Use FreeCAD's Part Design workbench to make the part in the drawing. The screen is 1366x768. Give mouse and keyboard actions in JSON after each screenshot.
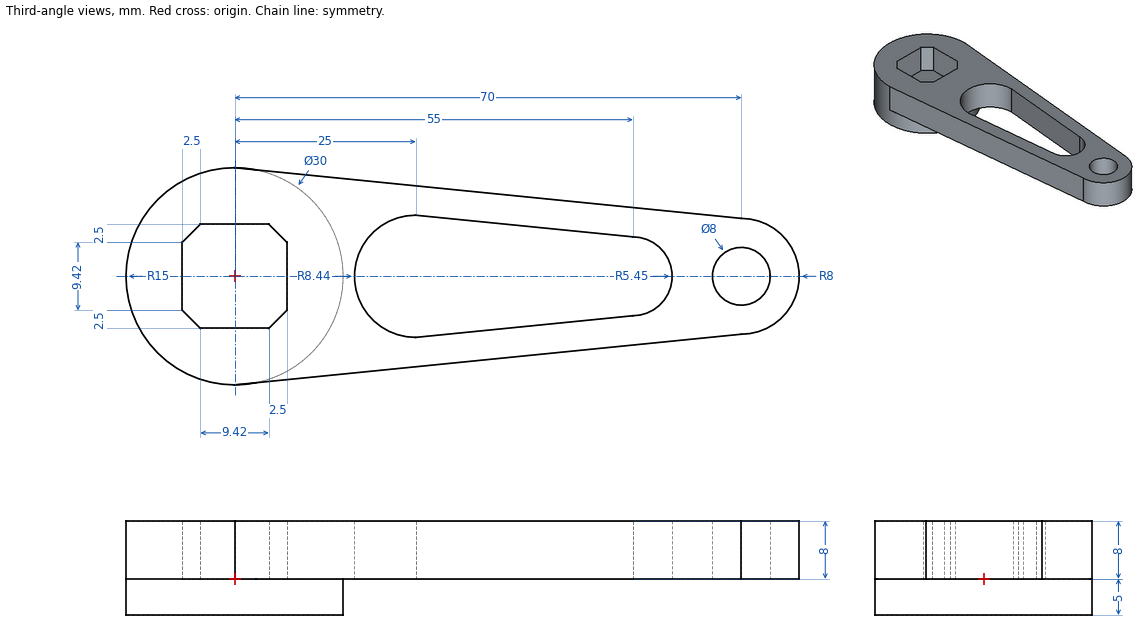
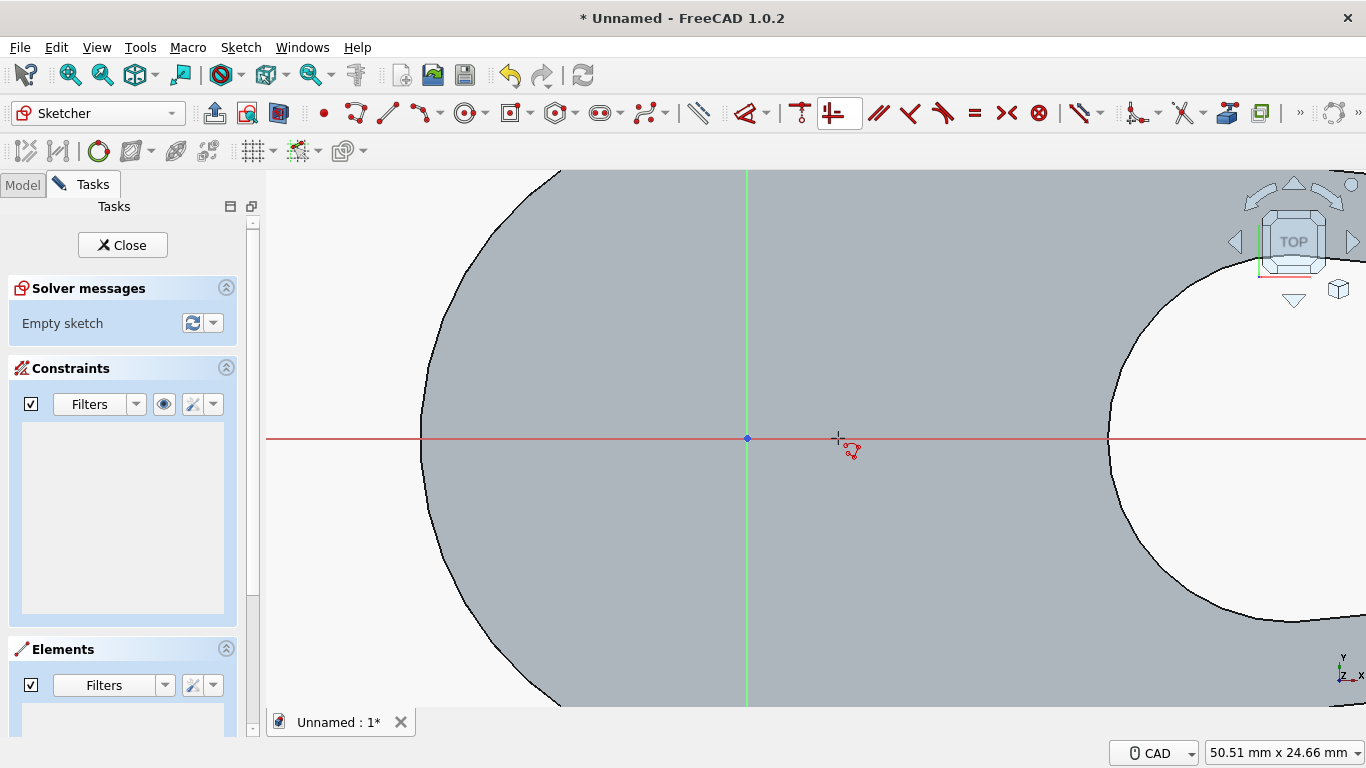
{"action": "left_click", "coordinate": [645, 281]}
{"action": "left_click", "coordinate": [590, 336]}
{"action": "left_click", "coordinate": [590, 541]}
{"action": "left_click", "coordinate": [645, 596]}
{"action": "left_click", "coordinate": [850, 596]}
{"action": "left_click", "coordinate": [904, 541]}
{"action": "left_click", "coordinate": [904, 336]}
{"action": "left_click", "coordinate": [850, 281]}
{"action": "left_click", "coordinate": [645, 282]}
{"action": "key", "text": "Escape"}
{"action": "key", "text": "Escape"}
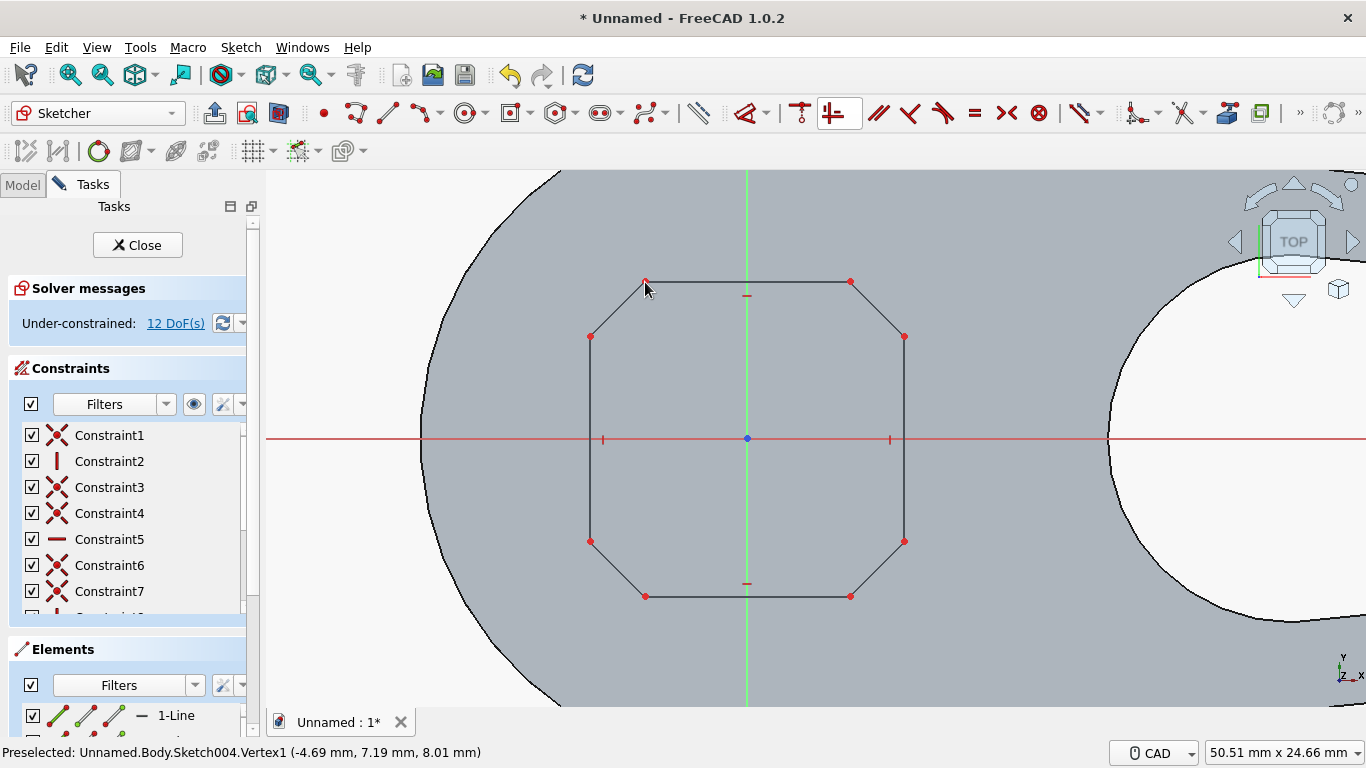
{"action": "left_click", "coordinate": [645, 282]}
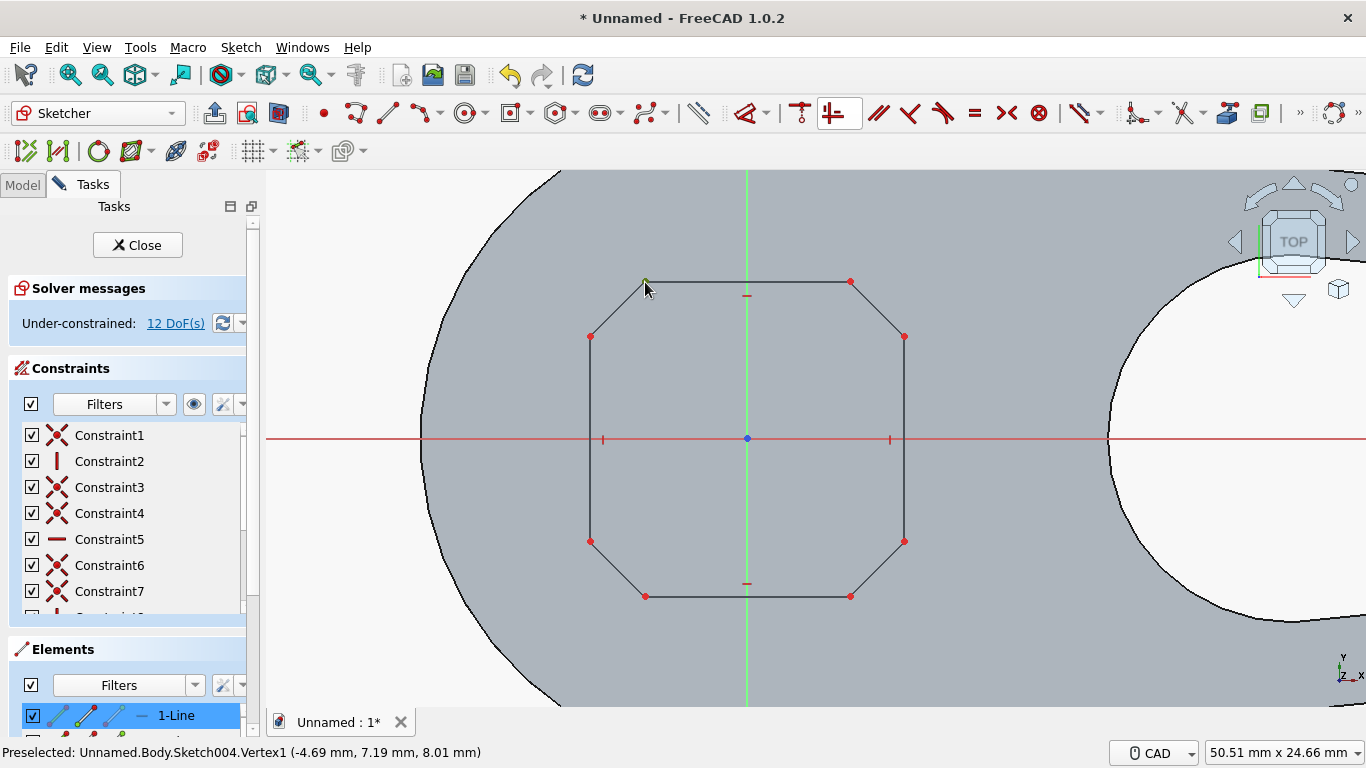
{"action": "left_click", "coordinate": [645, 597]}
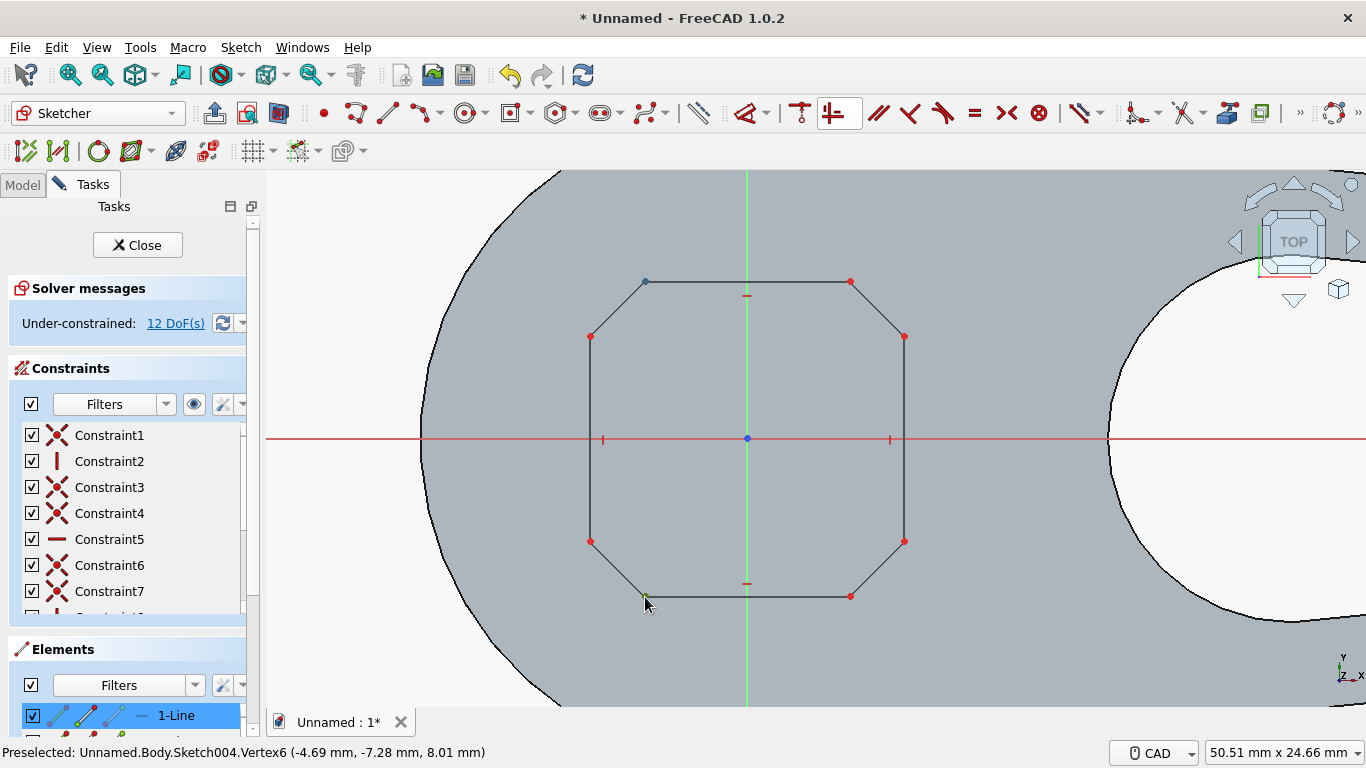
{"action": "left_click", "coordinate": [359, 438]}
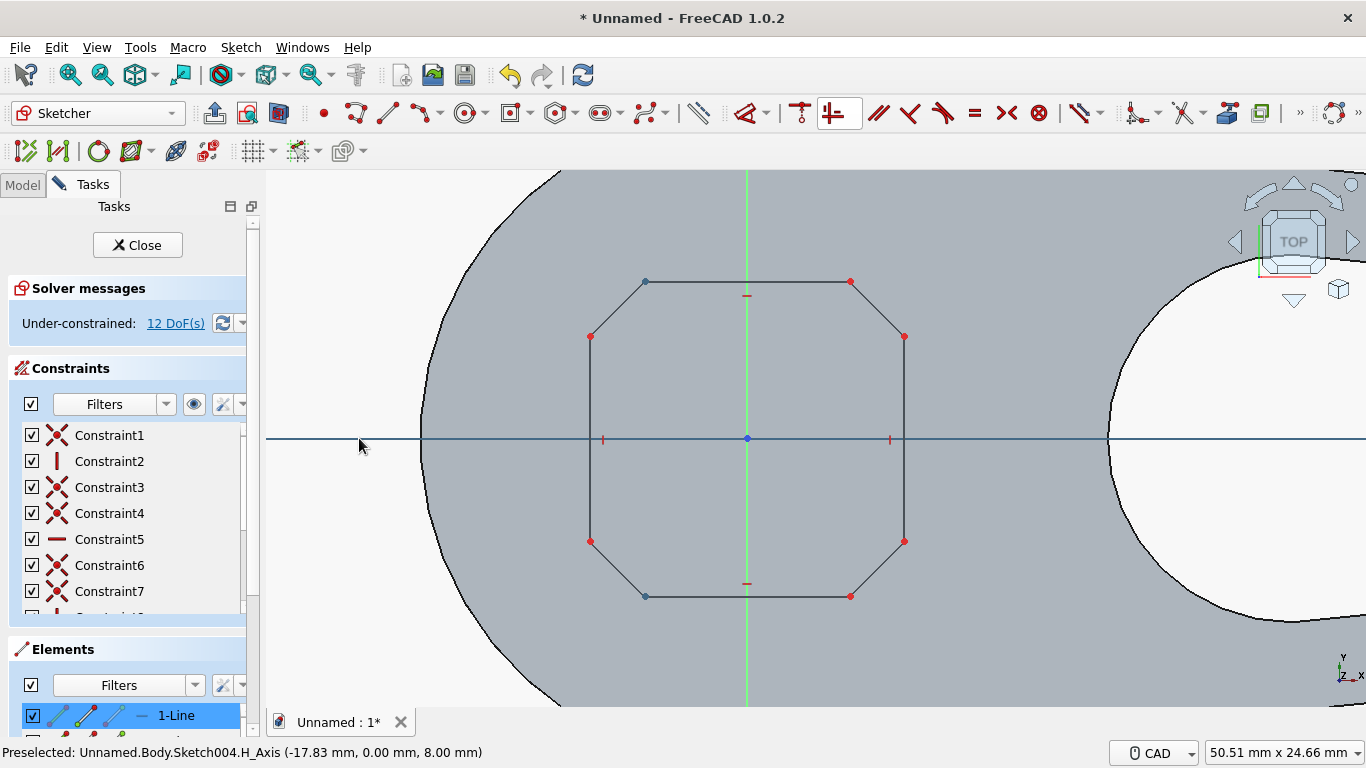
{"action": "key", "text": "s"}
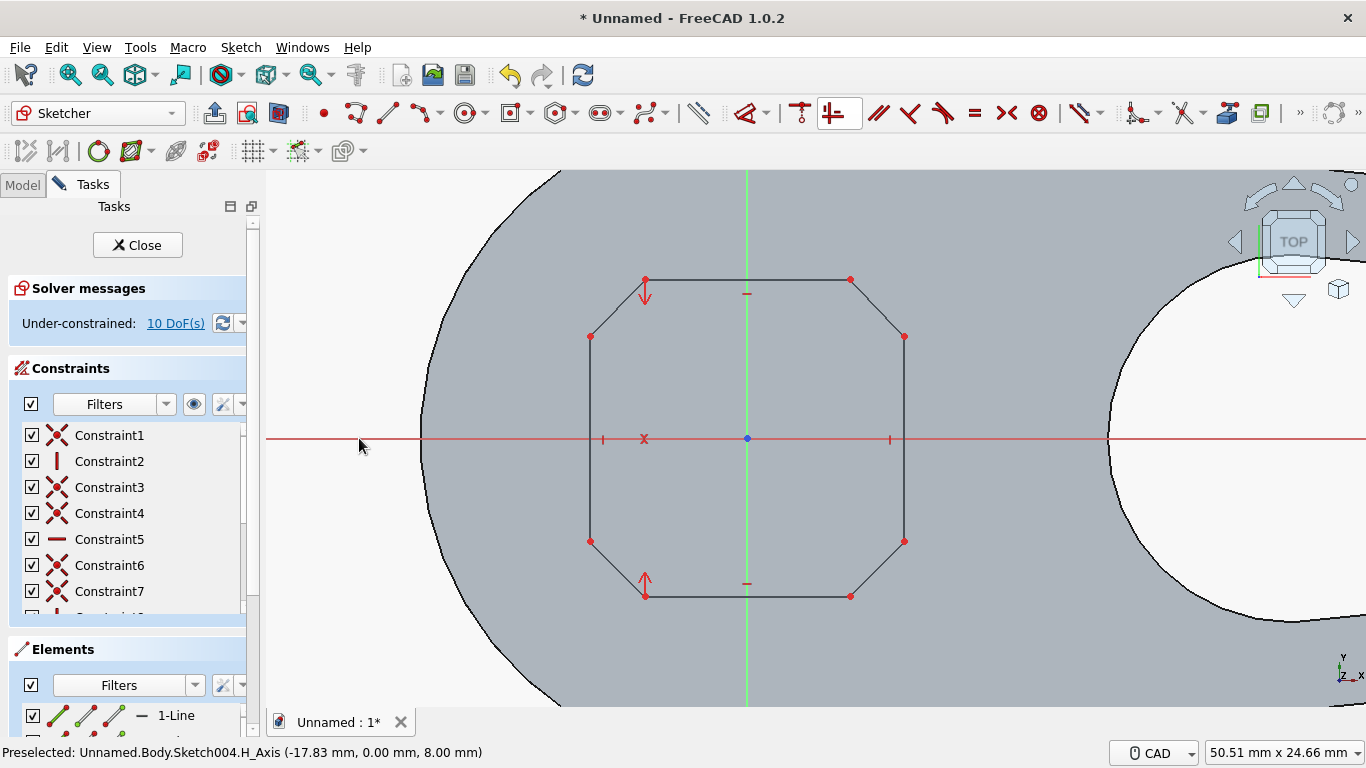
{"action": "left_click", "coordinate": [590, 542]}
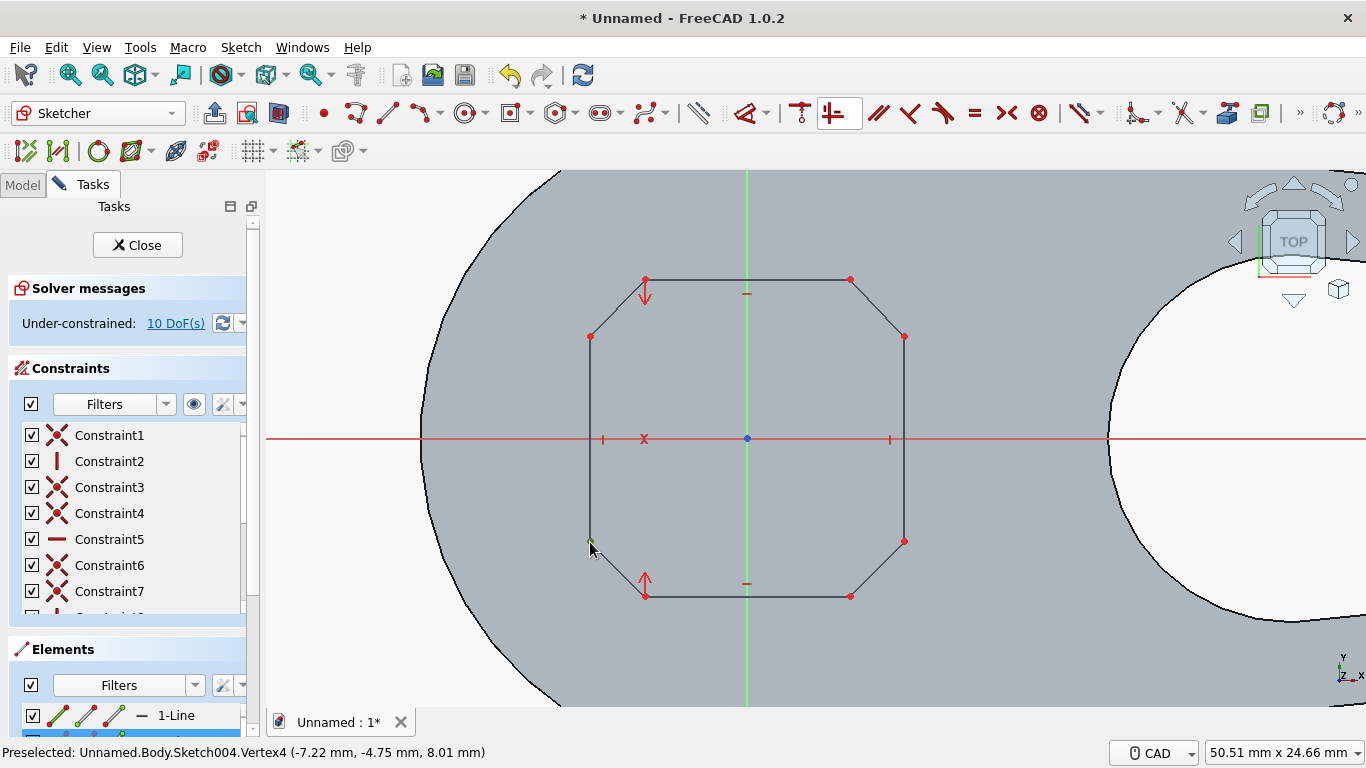
{"action": "left_click", "coordinate": [904, 542]}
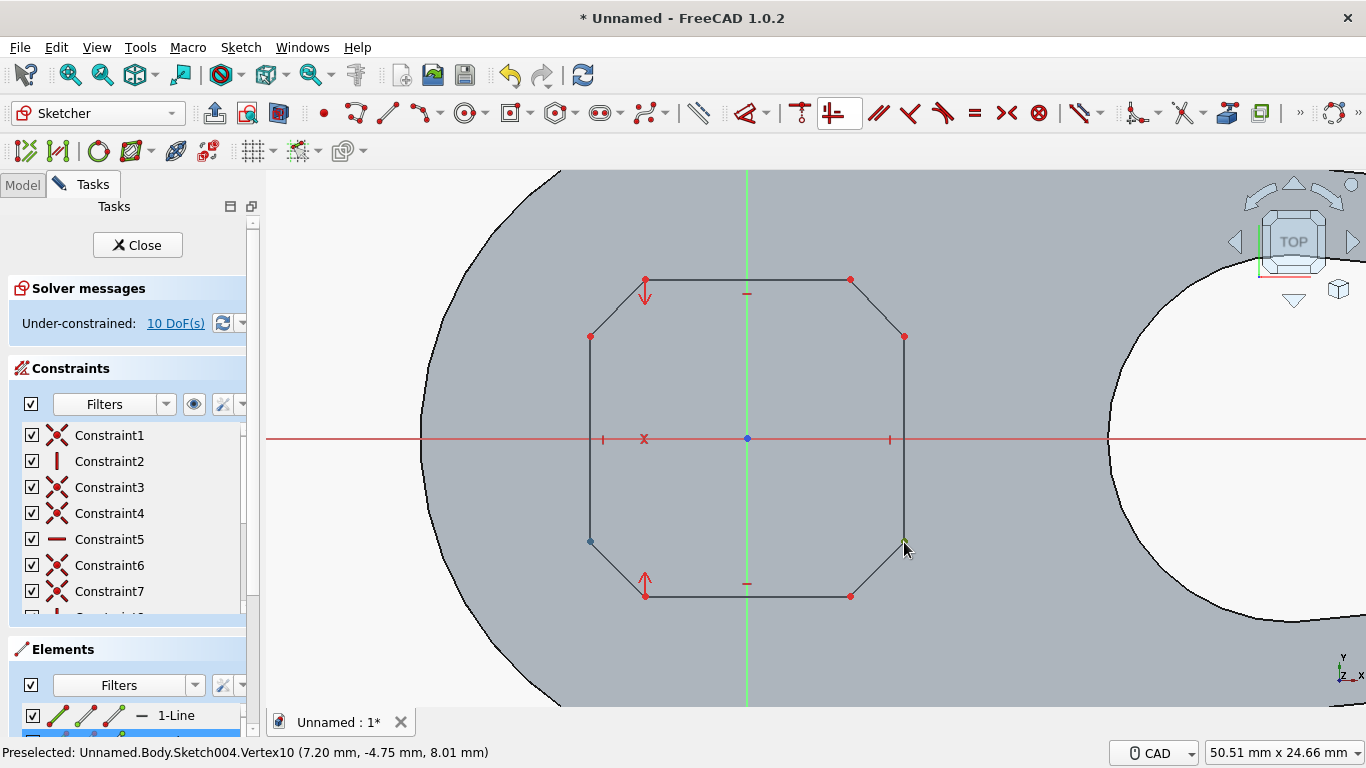
{"action": "left_click", "coordinate": [747, 645]}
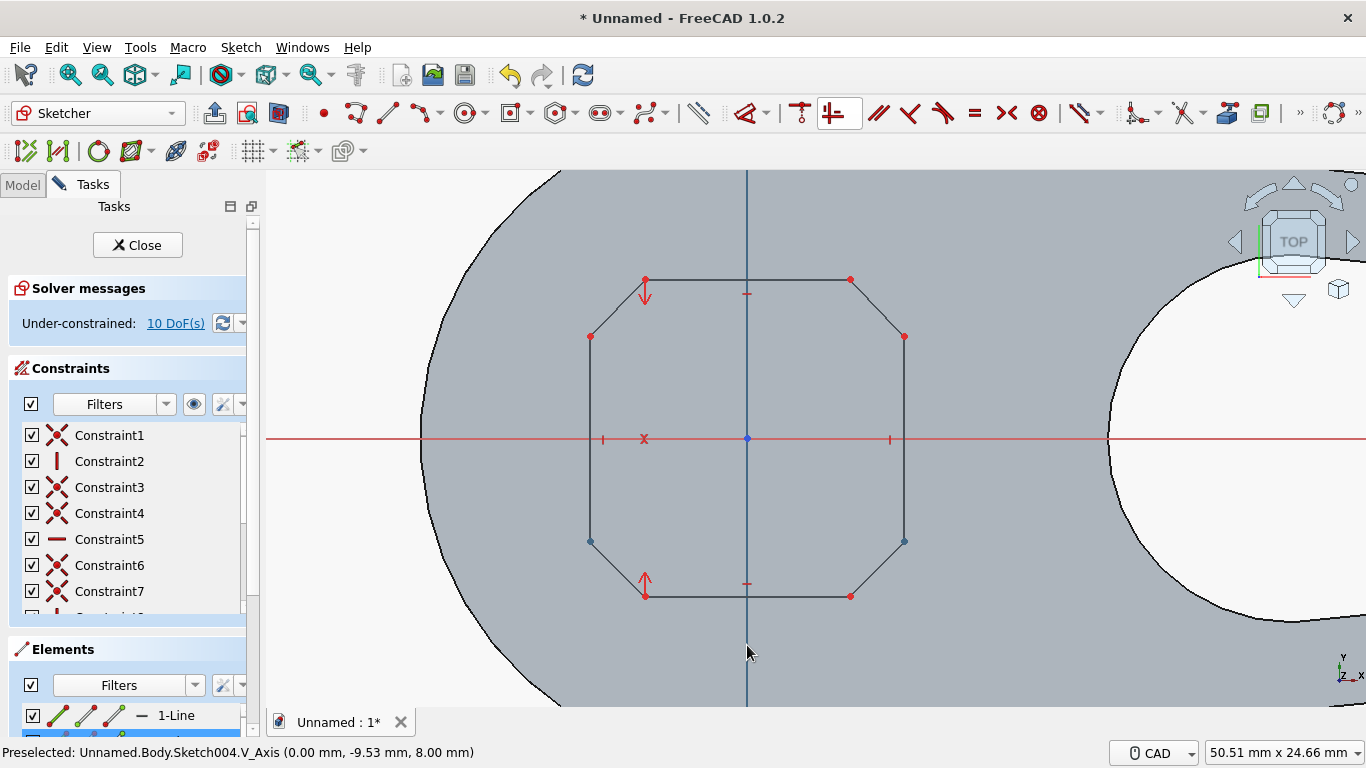
{"action": "left_click", "coordinate": [1008, 114]}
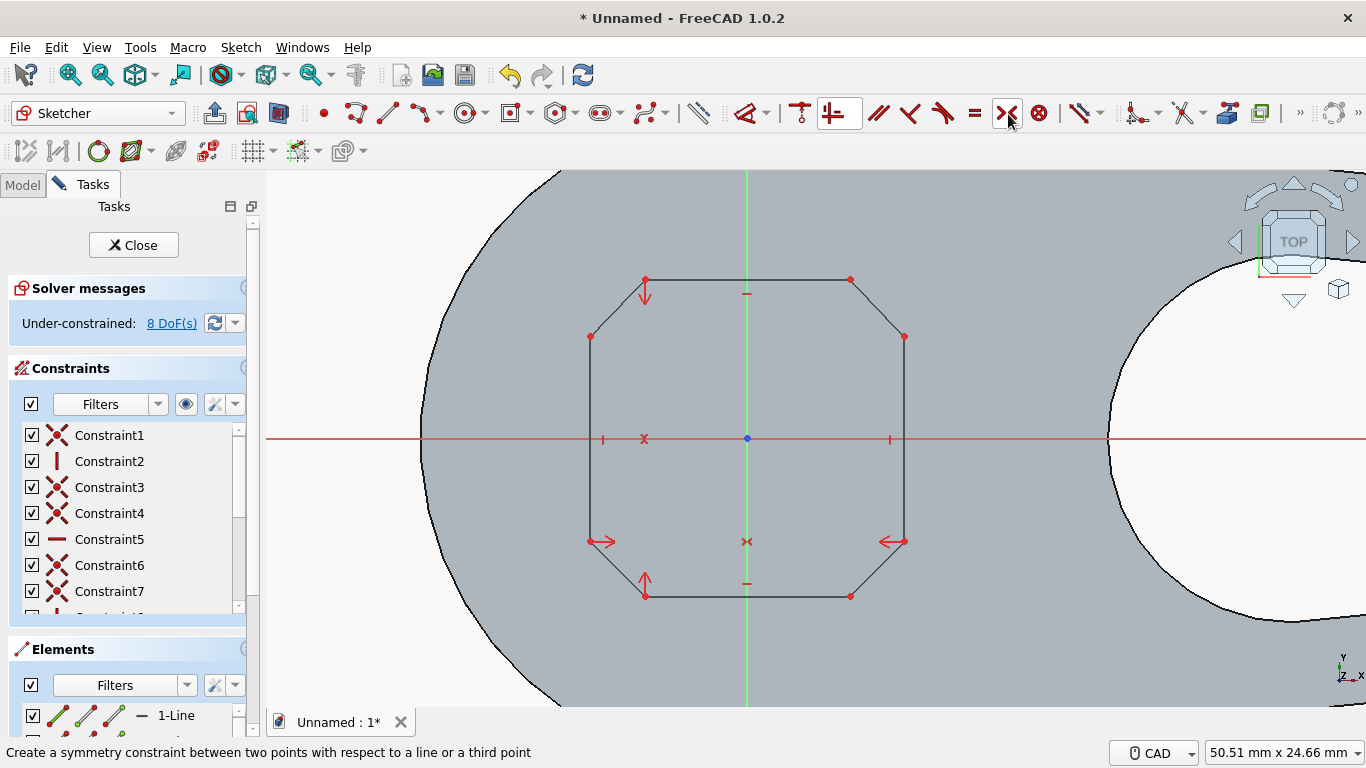
{"action": "left_click", "coordinate": [746, 114]}